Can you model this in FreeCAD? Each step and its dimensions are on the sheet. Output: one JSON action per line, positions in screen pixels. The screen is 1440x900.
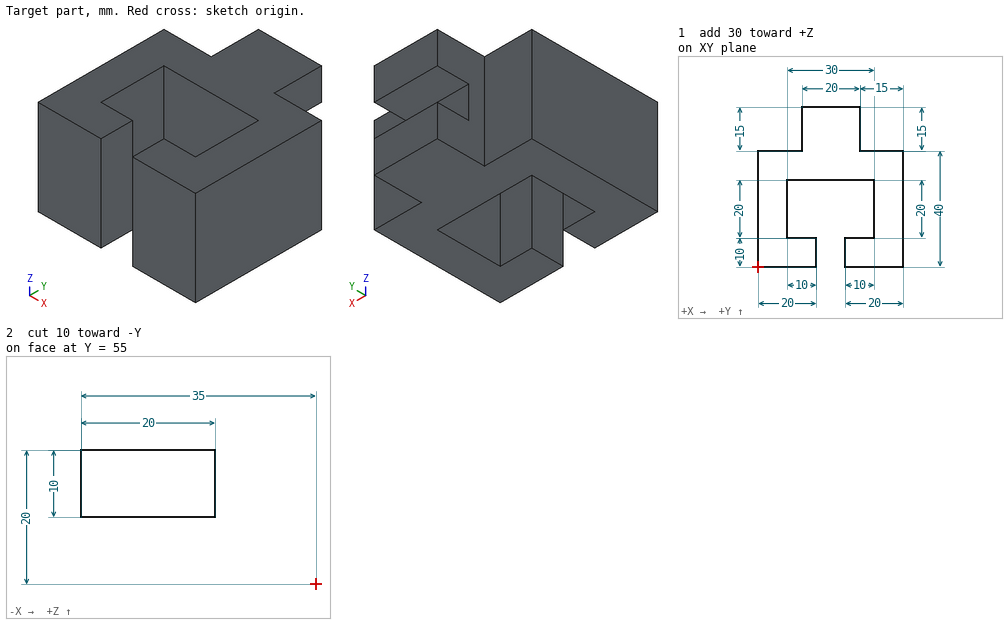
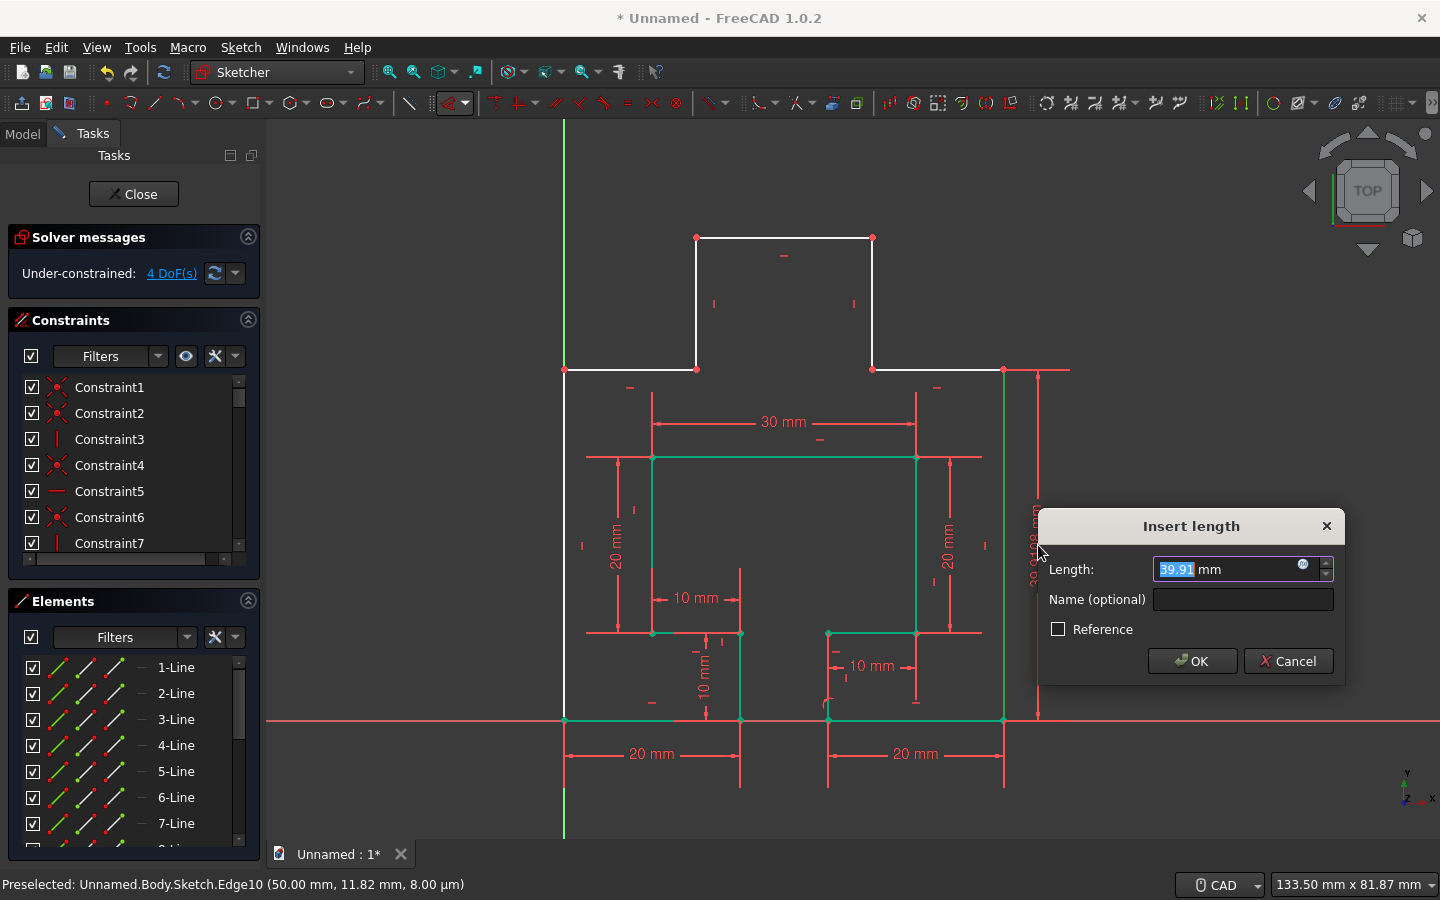
{"action": "type", "text": "40"}
{"action": "key", "text": "Return"}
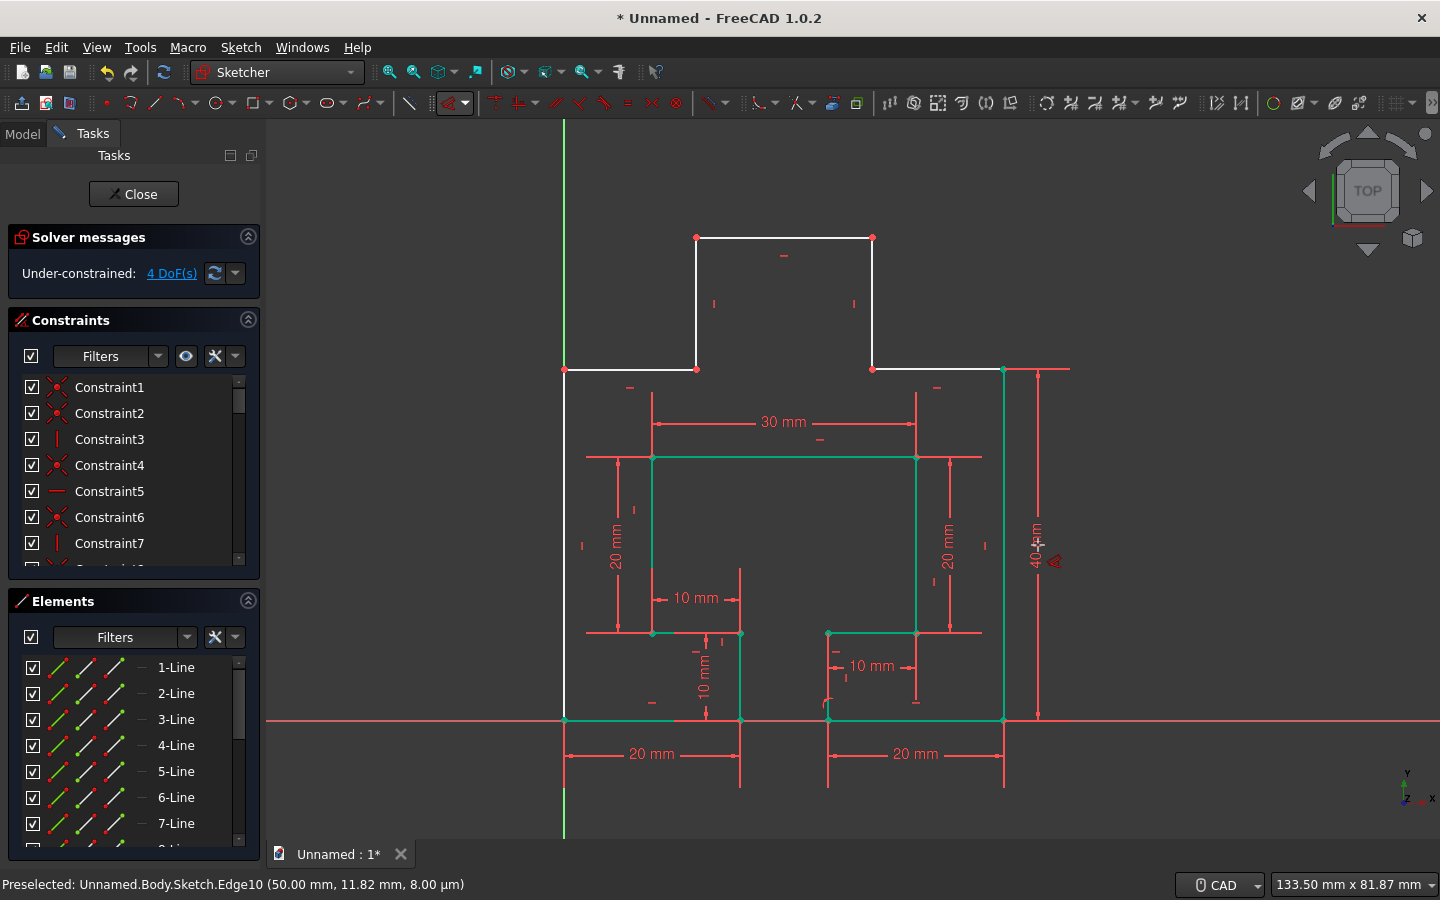
{"action": "left_click", "coordinate": [964, 369]}
{"action": "left_click", "coordinate": [938, 335]}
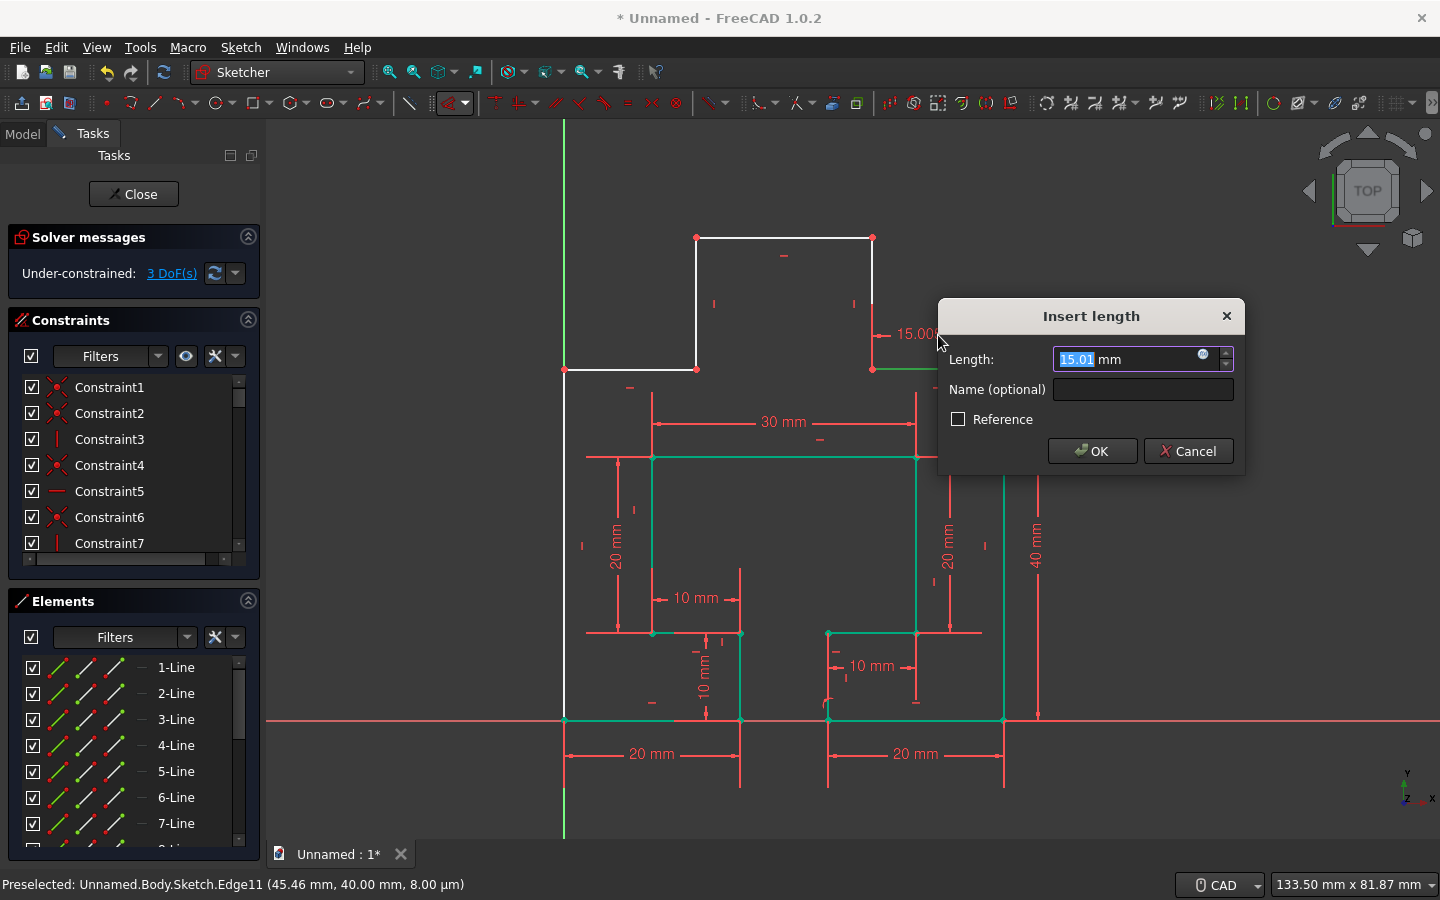
{"action": "type", "text": "15"}
{"action": "key", "text": "Return"}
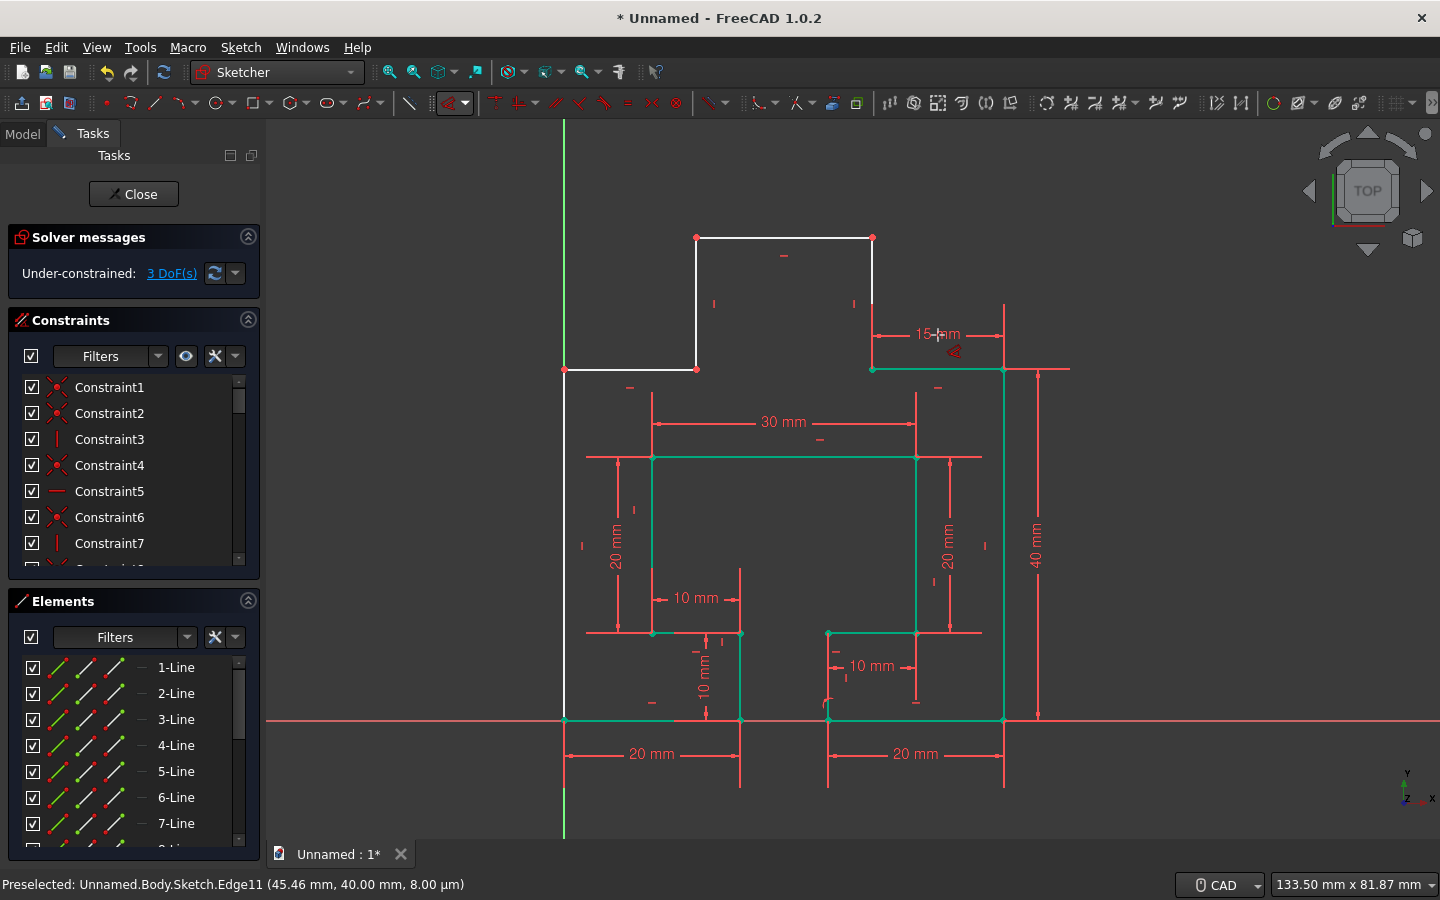
{"action": "left_click", "coordinate": [872, 330]}
{"action": "left_click", "coordinate": [906, 304]}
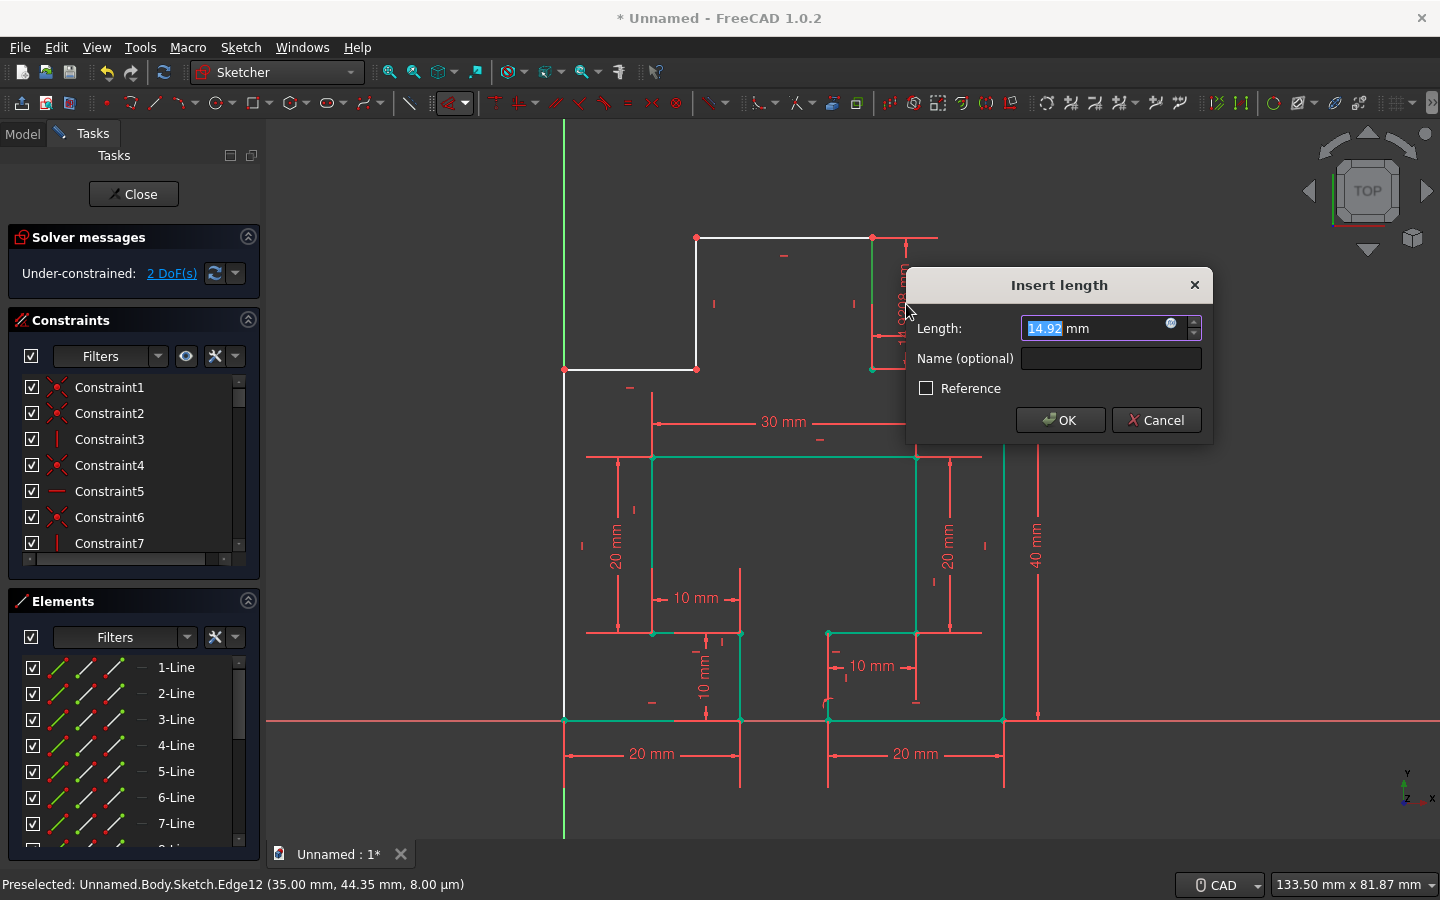
{"action": "type", "text": "15"}
{"action": "key", "text": "Return"}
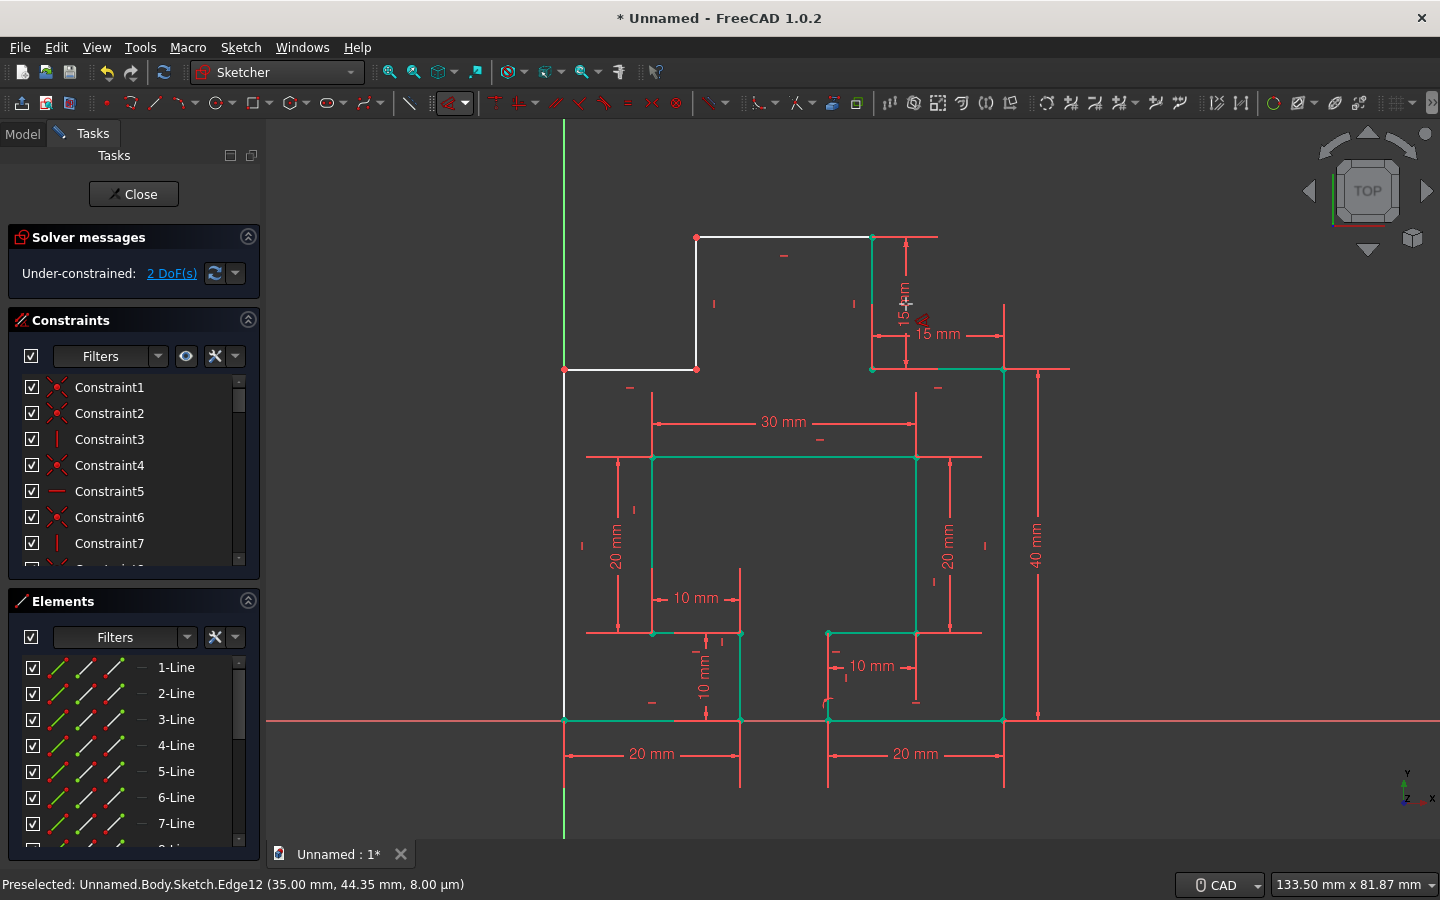
{"action": "left_click", "coordinate": [819, 237]}
{"action": "left_click", "coordinate": [784, 203]}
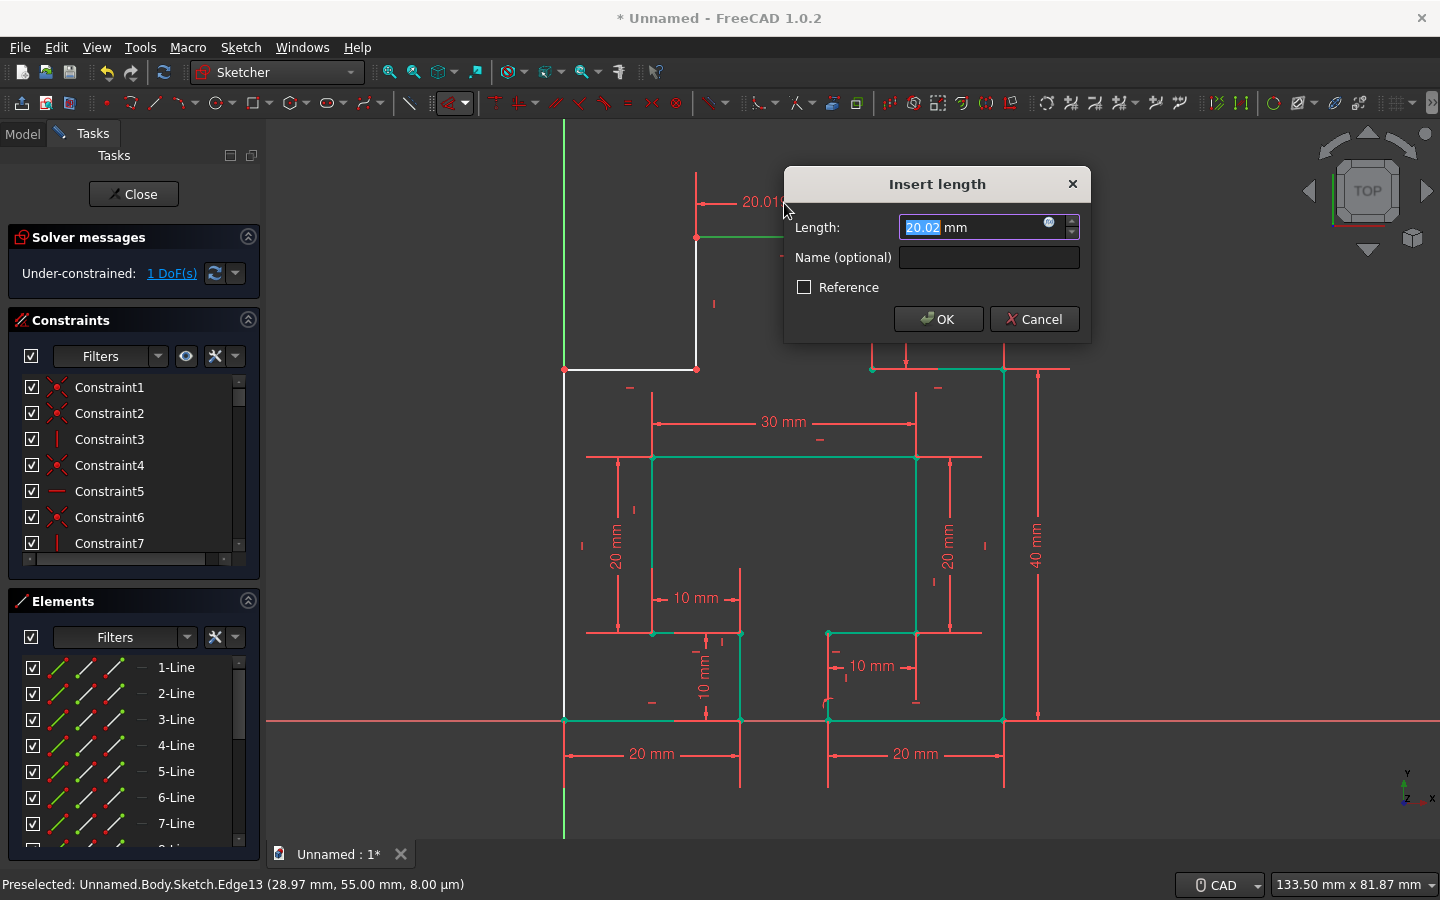
{"action": "type", "text": "20"}
{"action": "key", "text": "Return"}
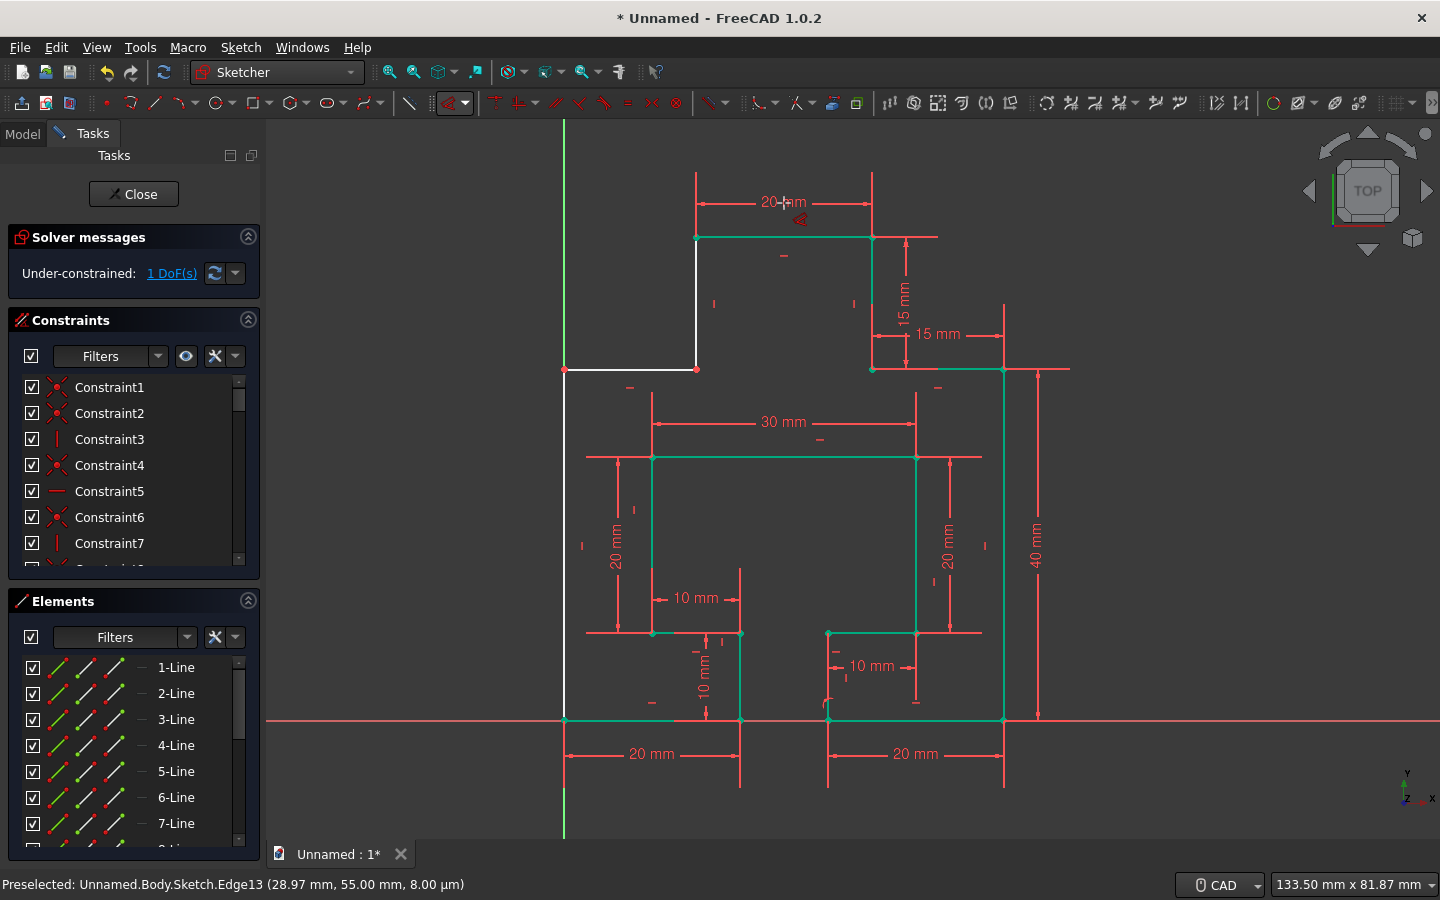
{"action": "left_click", "coordinate": [696, 277]}
{"action": "left_click", "coordinate": [662, 304]}